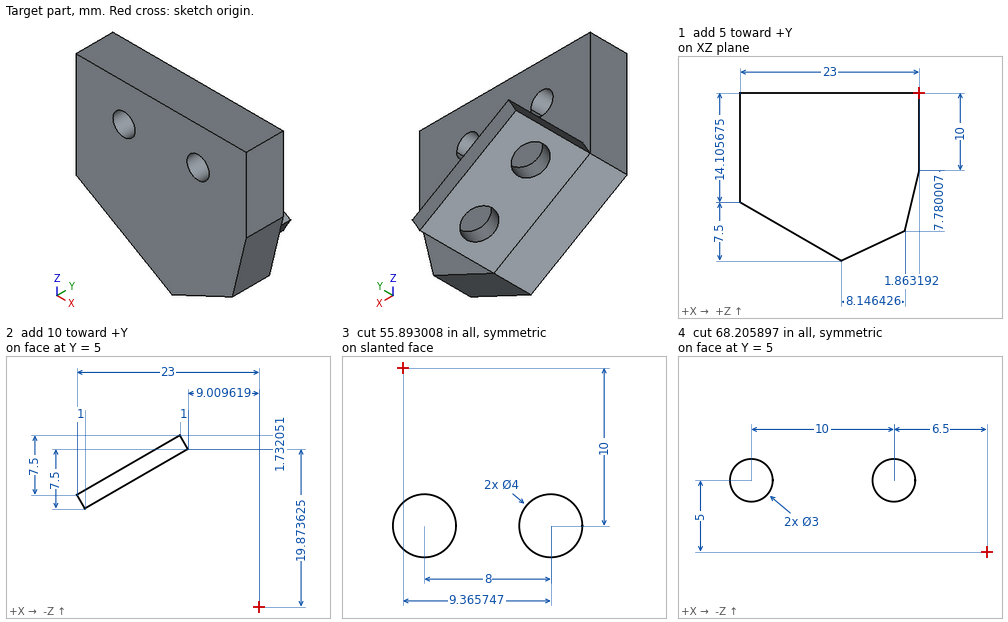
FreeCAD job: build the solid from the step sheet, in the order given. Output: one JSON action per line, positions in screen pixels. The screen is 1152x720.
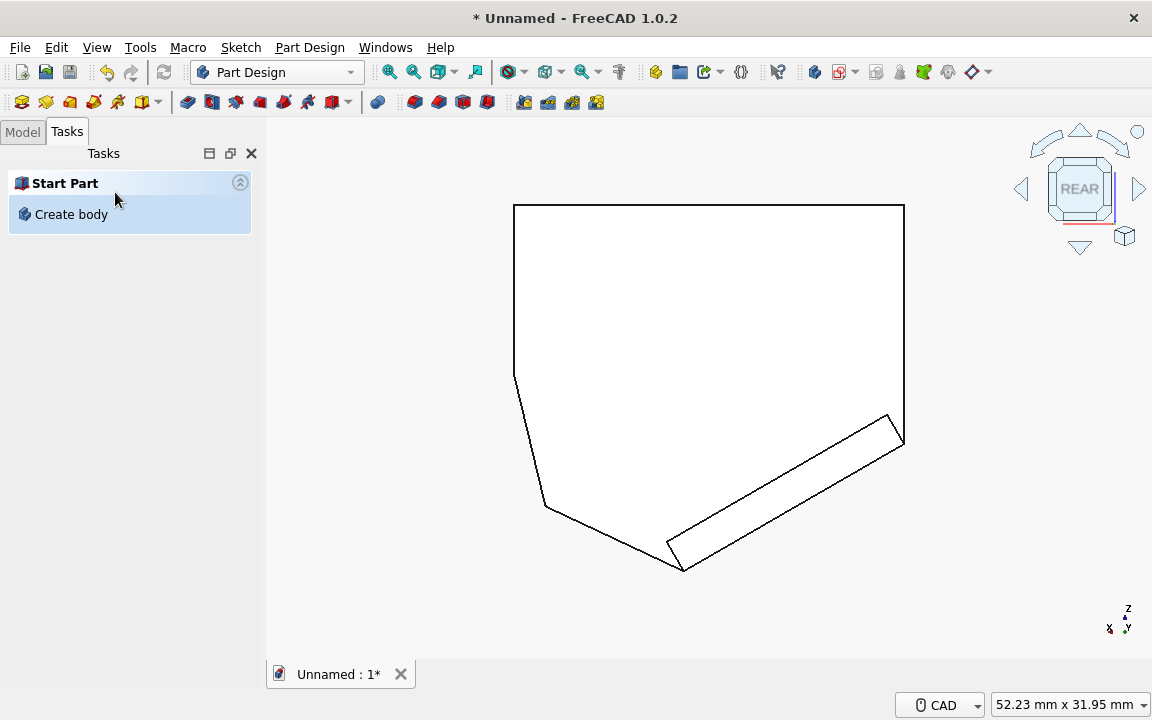
{"action": "key", "text": "0"}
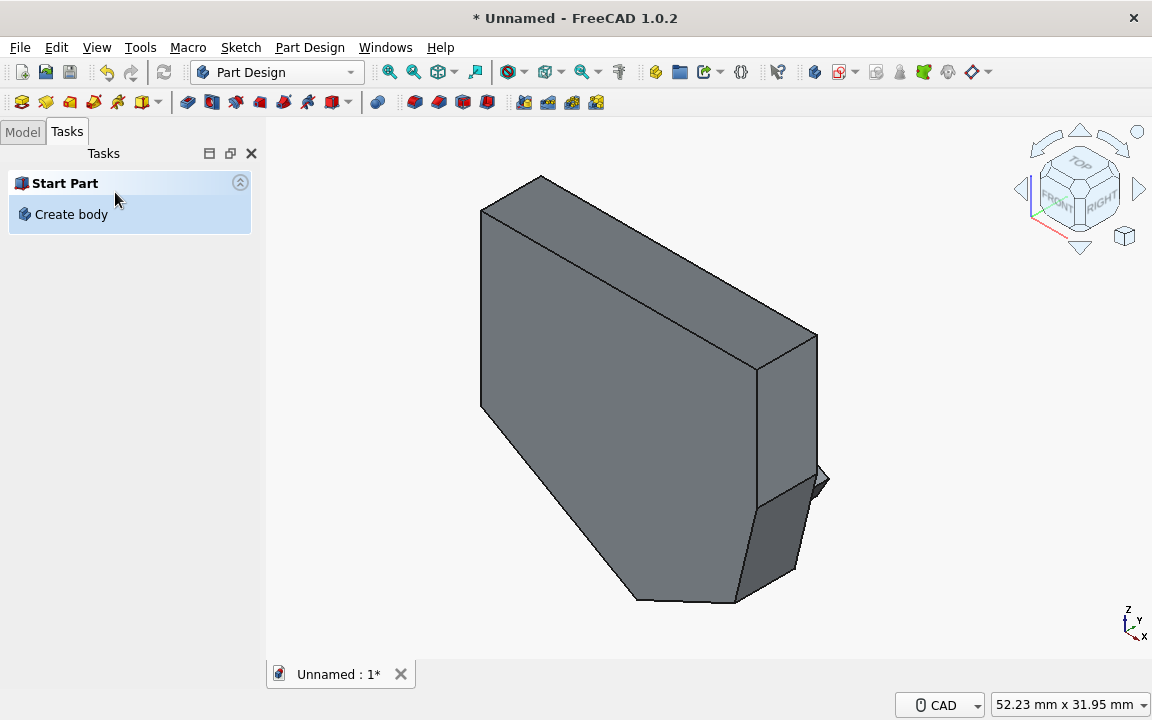
{"action": "key", "text": "v f"}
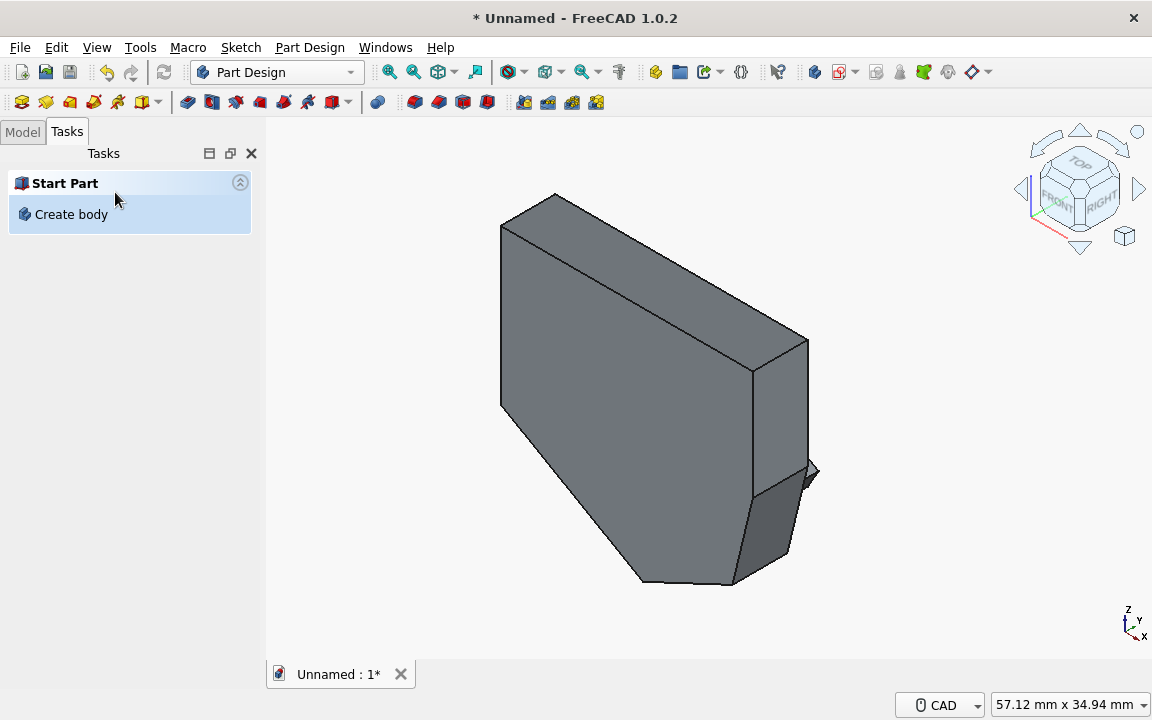
{"action": "key", "text": "2"}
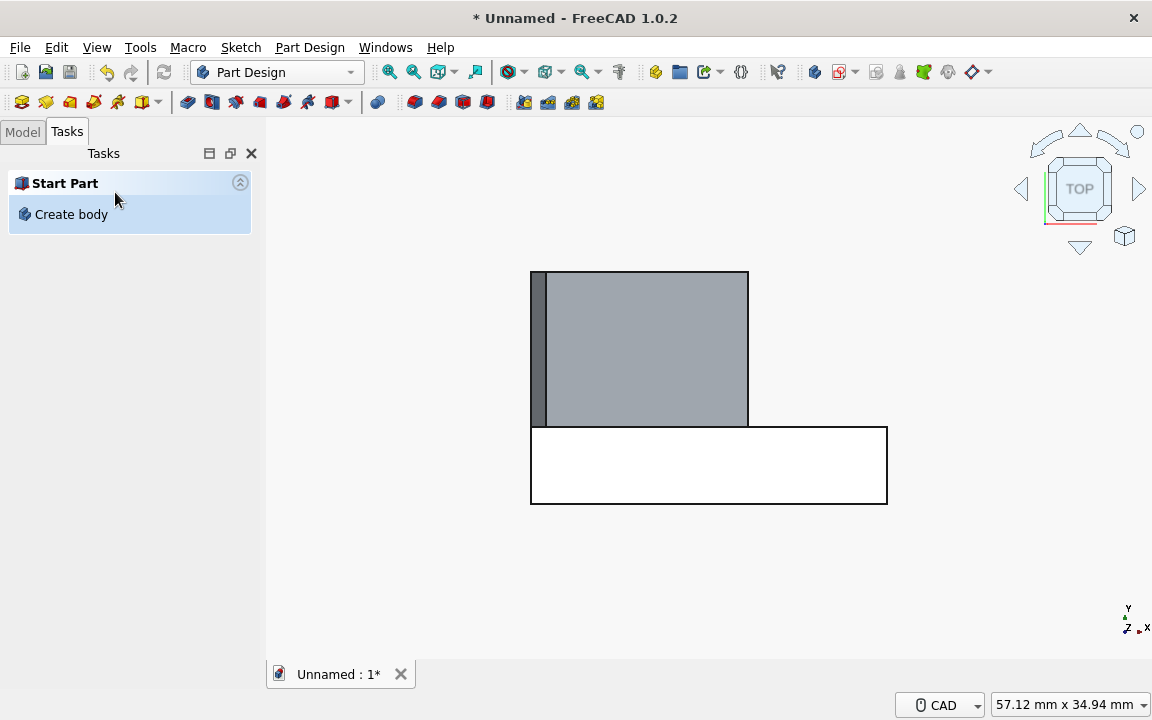
{"action": "left_click", "coordinate": [390, 72]}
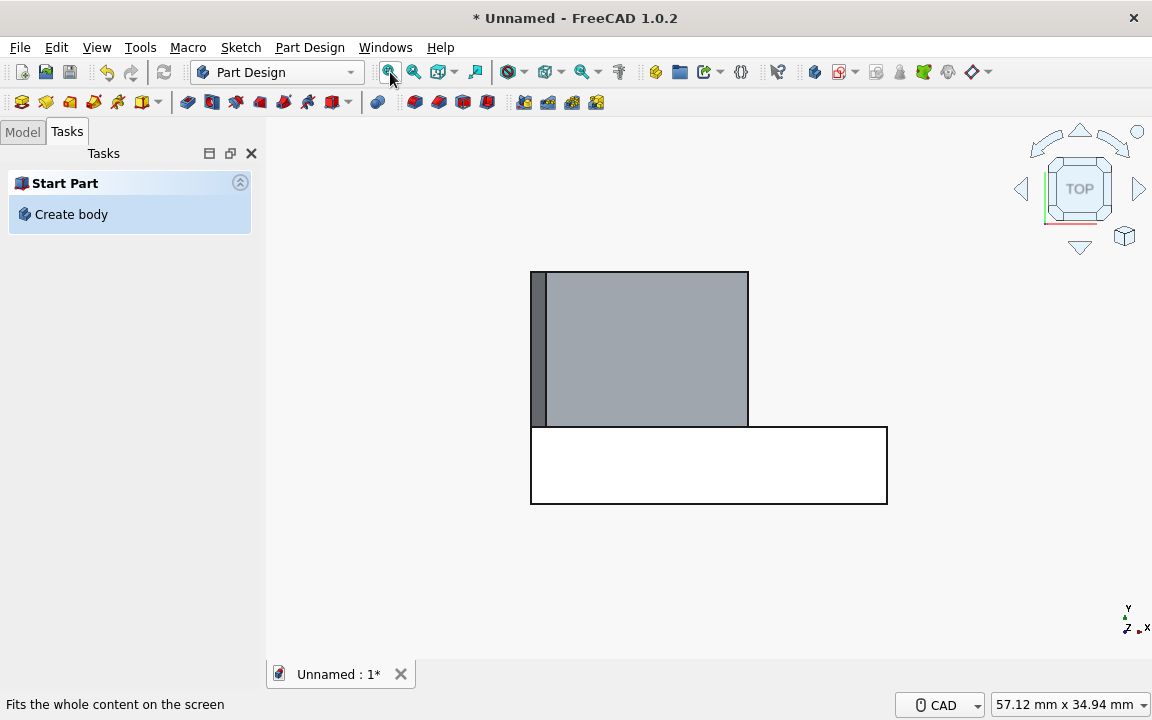
{"action": "left_click", "coordinate": [676, 348]}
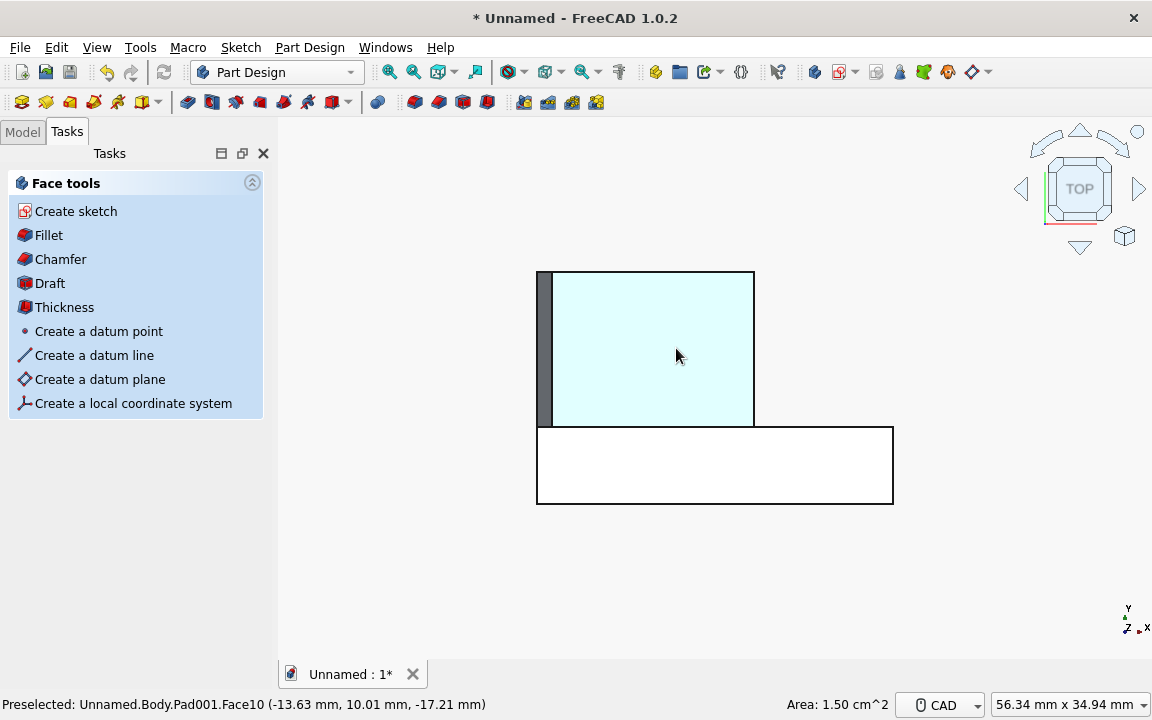
{"action": "left_click", "coordinate": [840, 72]}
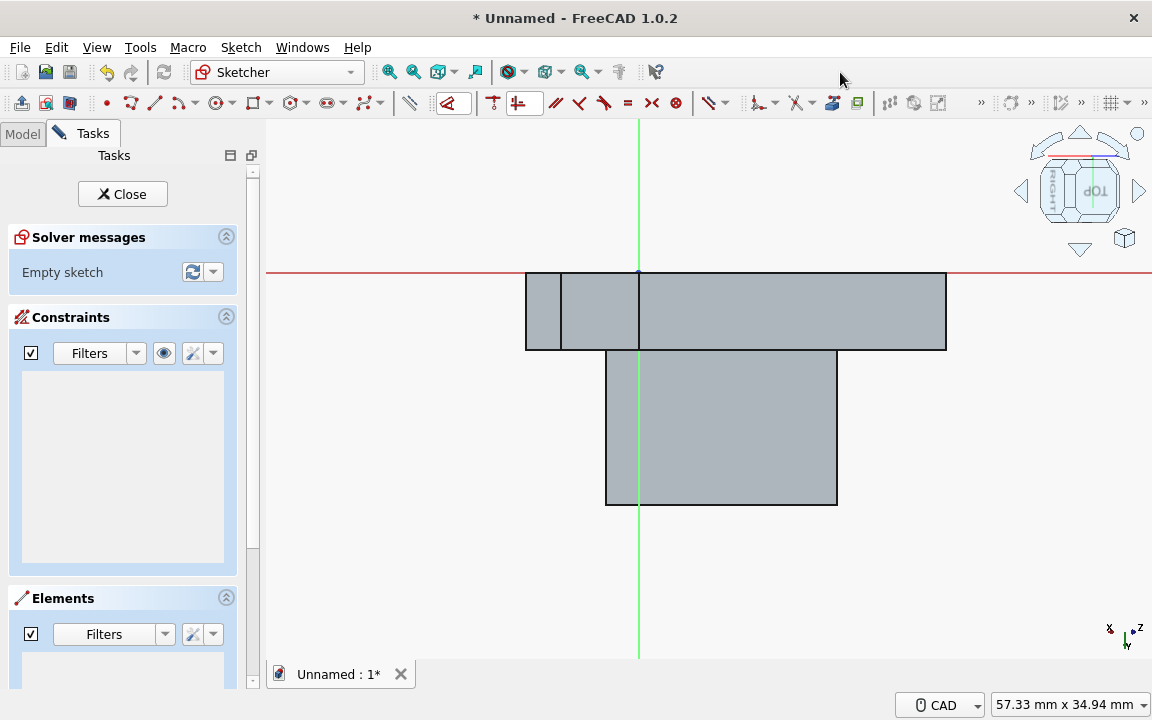
{"action": "scroll", "coordinate": [820, 338], "scroll_direction": "up", "scroll_amount": 3}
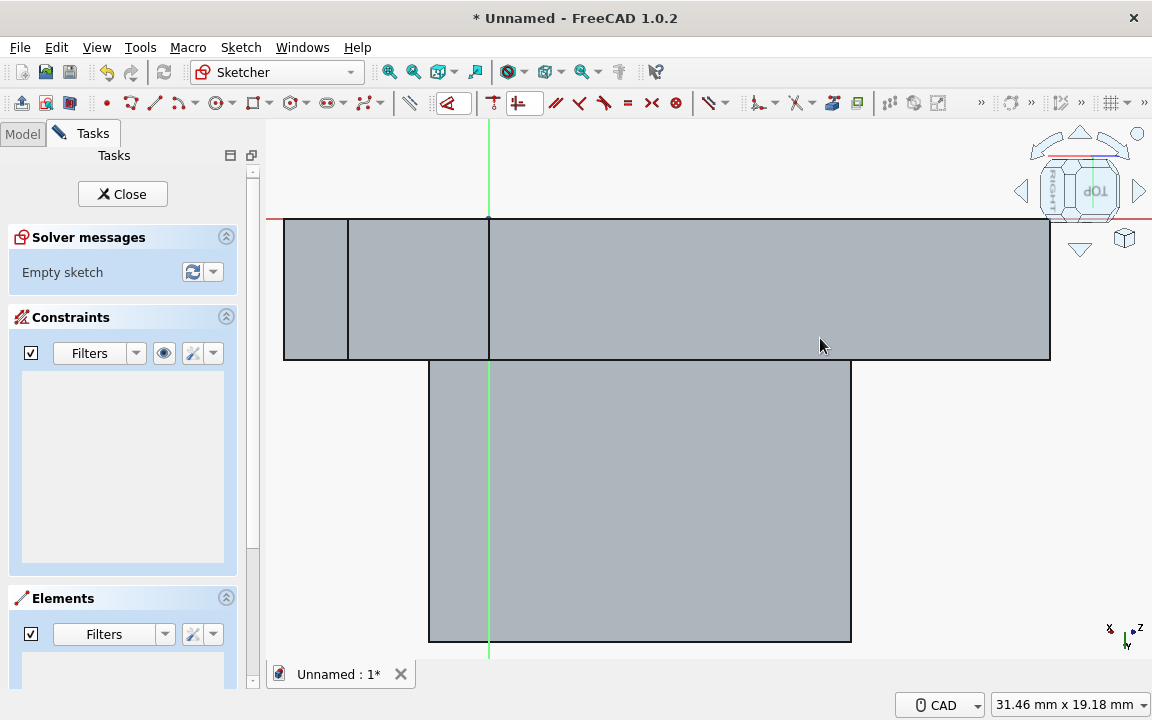
{"action": "left_click", "coordinate": [216, 104]}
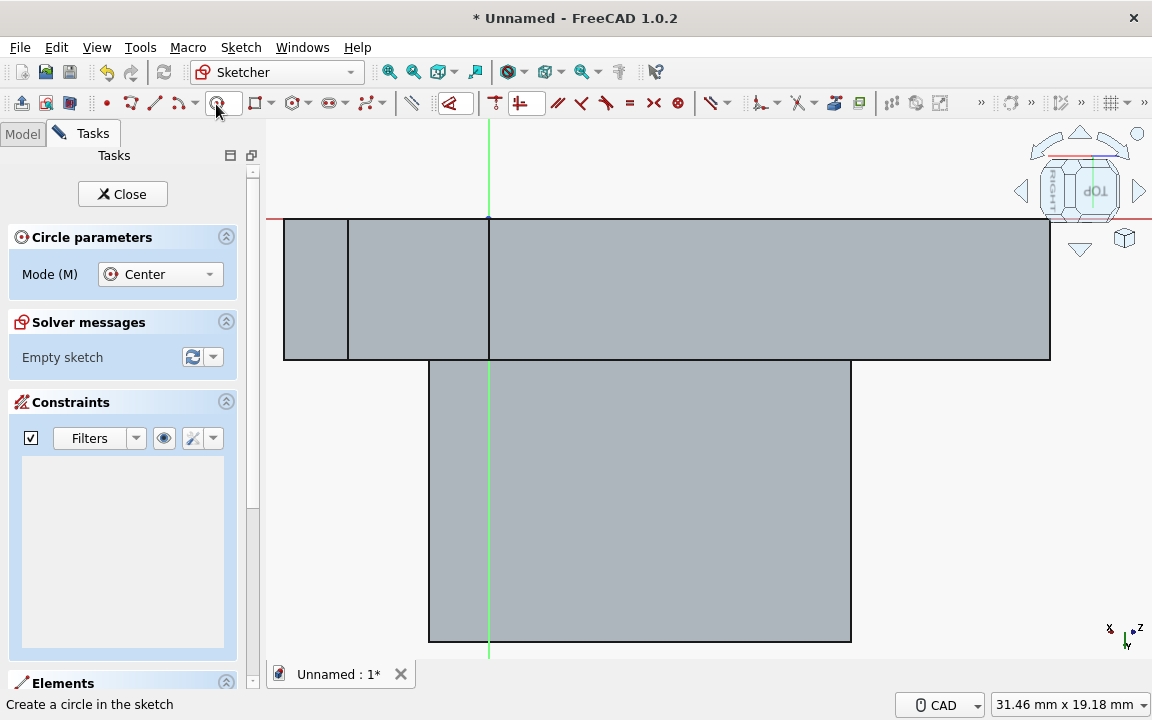
{"action": "left_click", "coordinate": [753, 501]}
{"action": "mouse_move", "coordinate": [792, 461]}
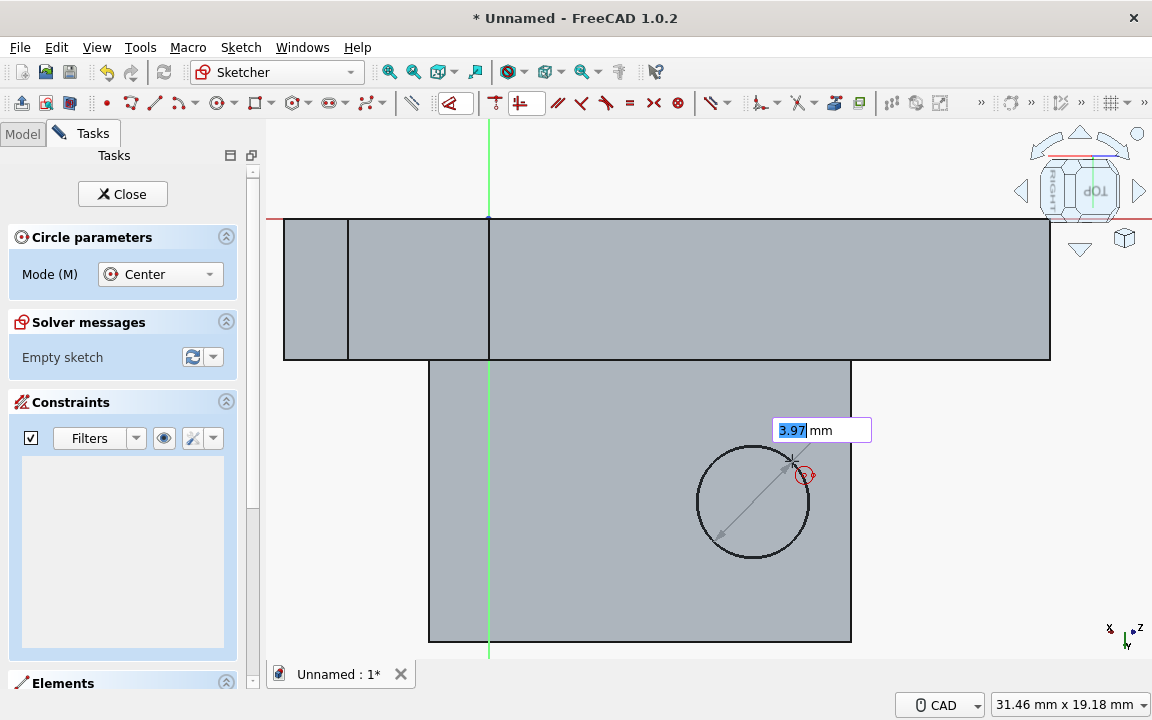
{"action": "type", "text": "4"}
{"action": "key", "text": "Return"}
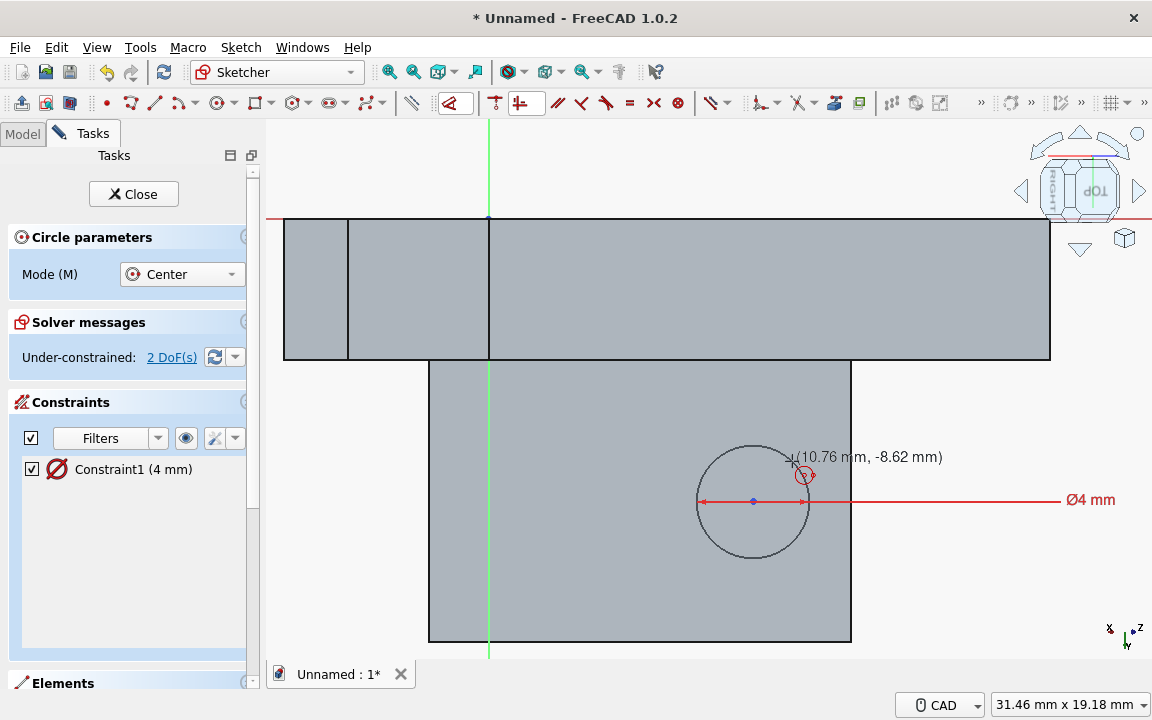
{"action": "left_click", "coordinate": [527, 501]}
{"action": "mouse_move", "coordinate": [567, 461]}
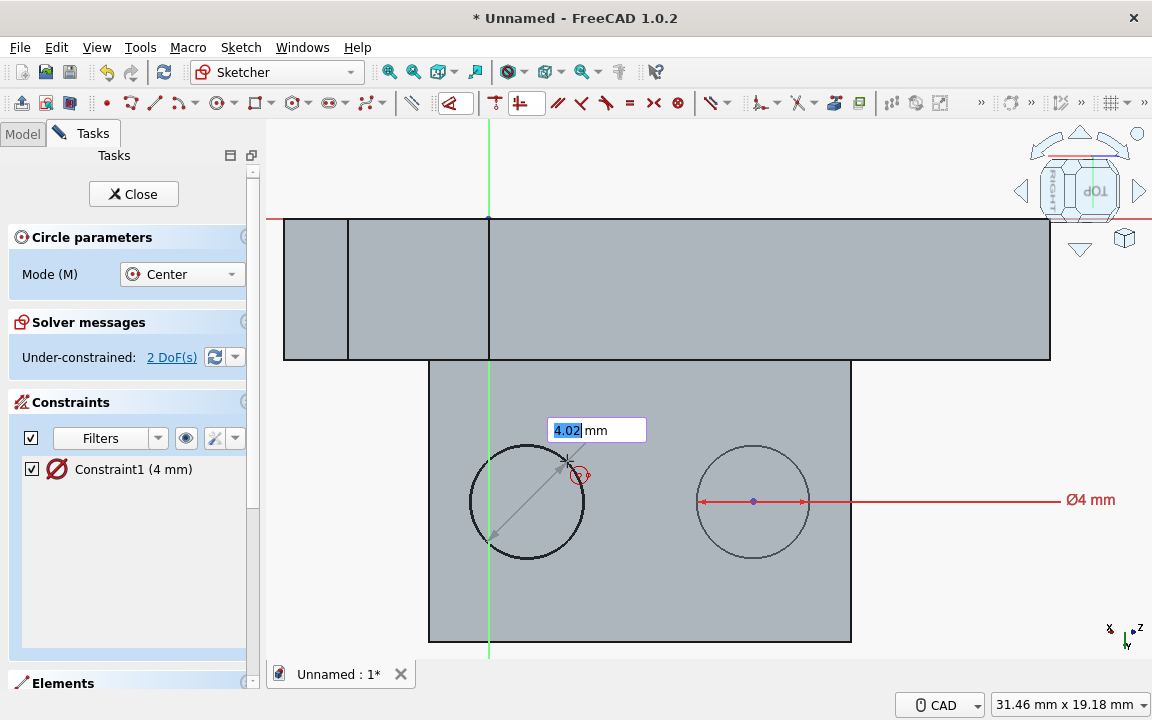
{"action": "type", "text": "4"}
{"action": "key", "text": "Return"}
{"action": "key", "text": "Escape"}